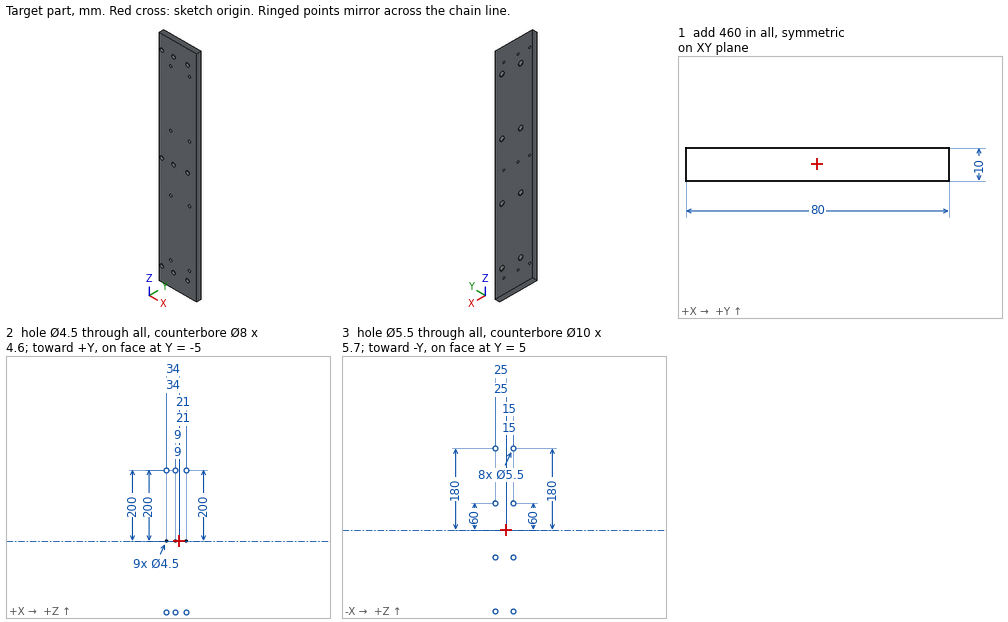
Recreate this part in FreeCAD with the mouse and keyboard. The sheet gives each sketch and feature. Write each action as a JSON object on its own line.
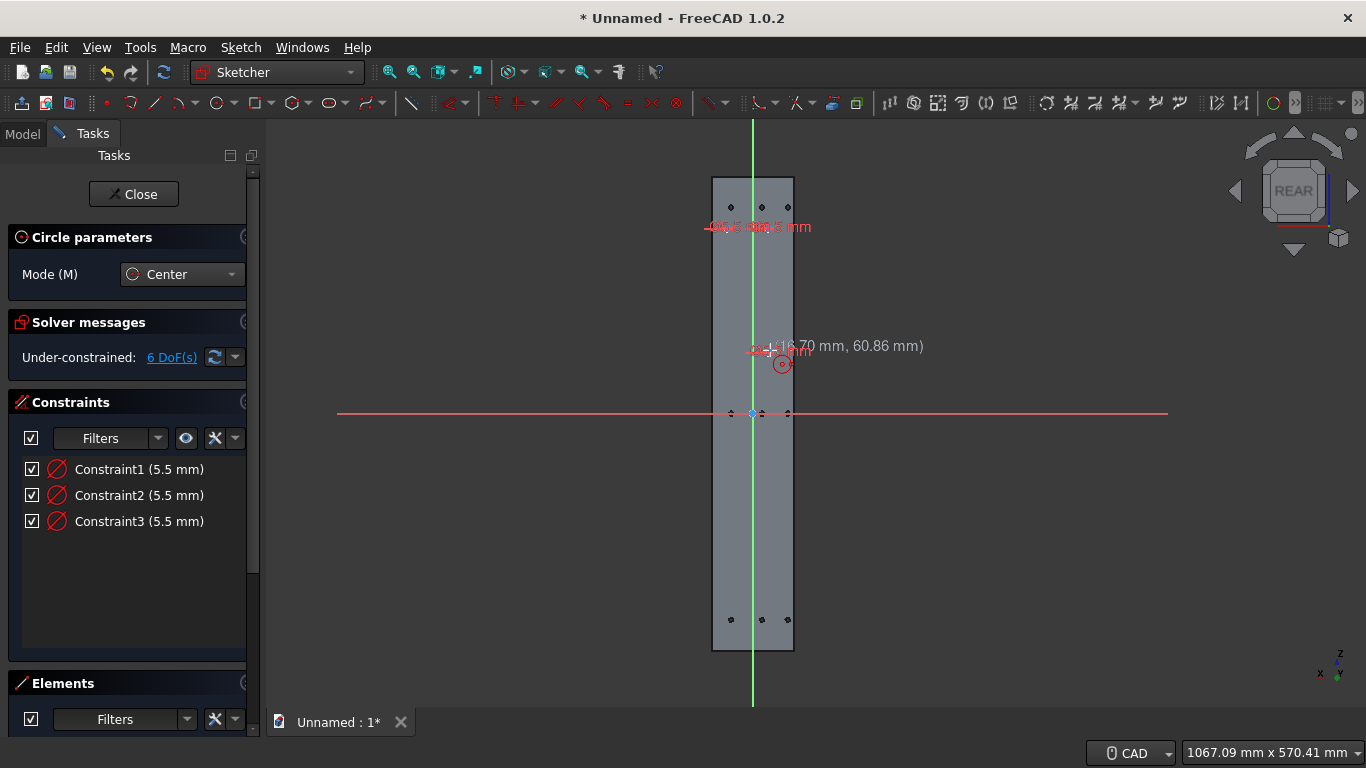
{"action": "scroll", "coordinate": [727, 352], "scroll_direction": "up", "scroll_amount": 11}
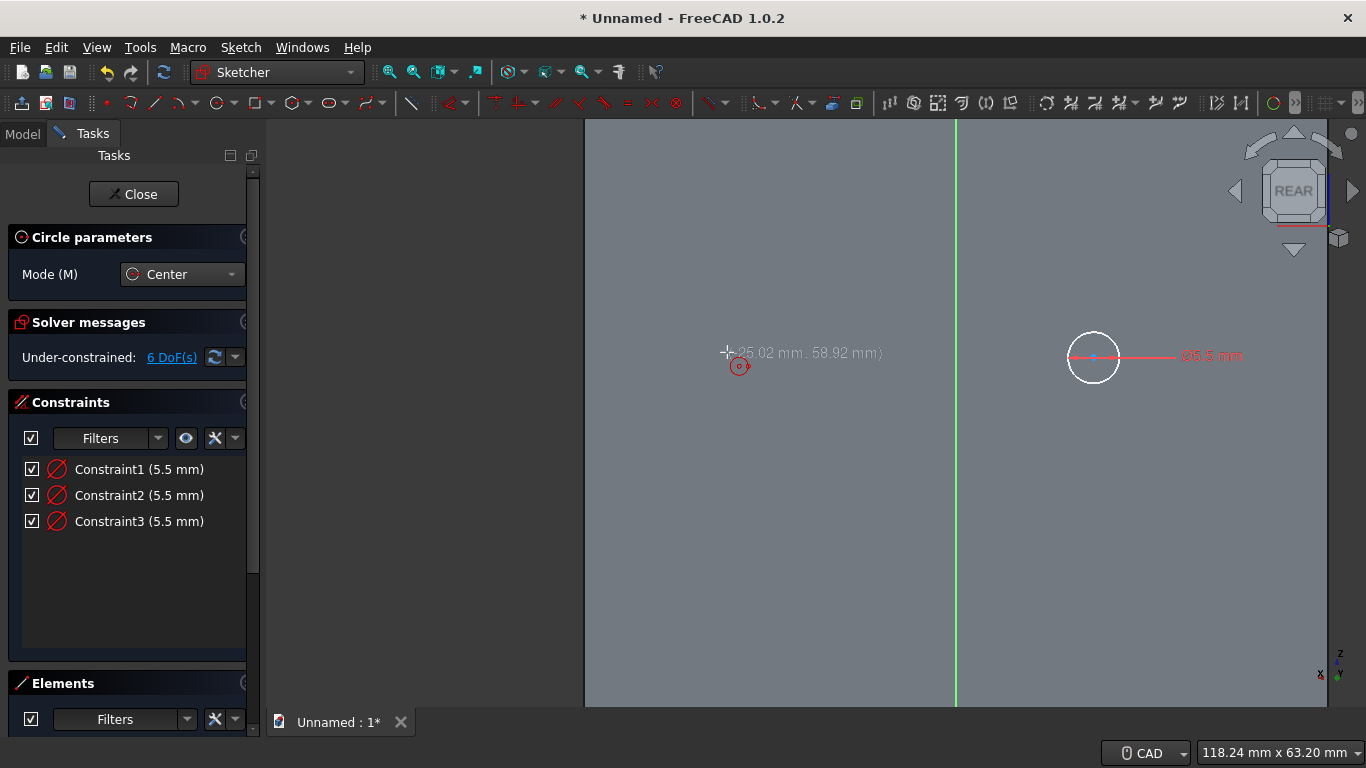
{"action": "scroll", "coordinate": [727, 352], "scroll_direction": "down", "scroll_amount": 11}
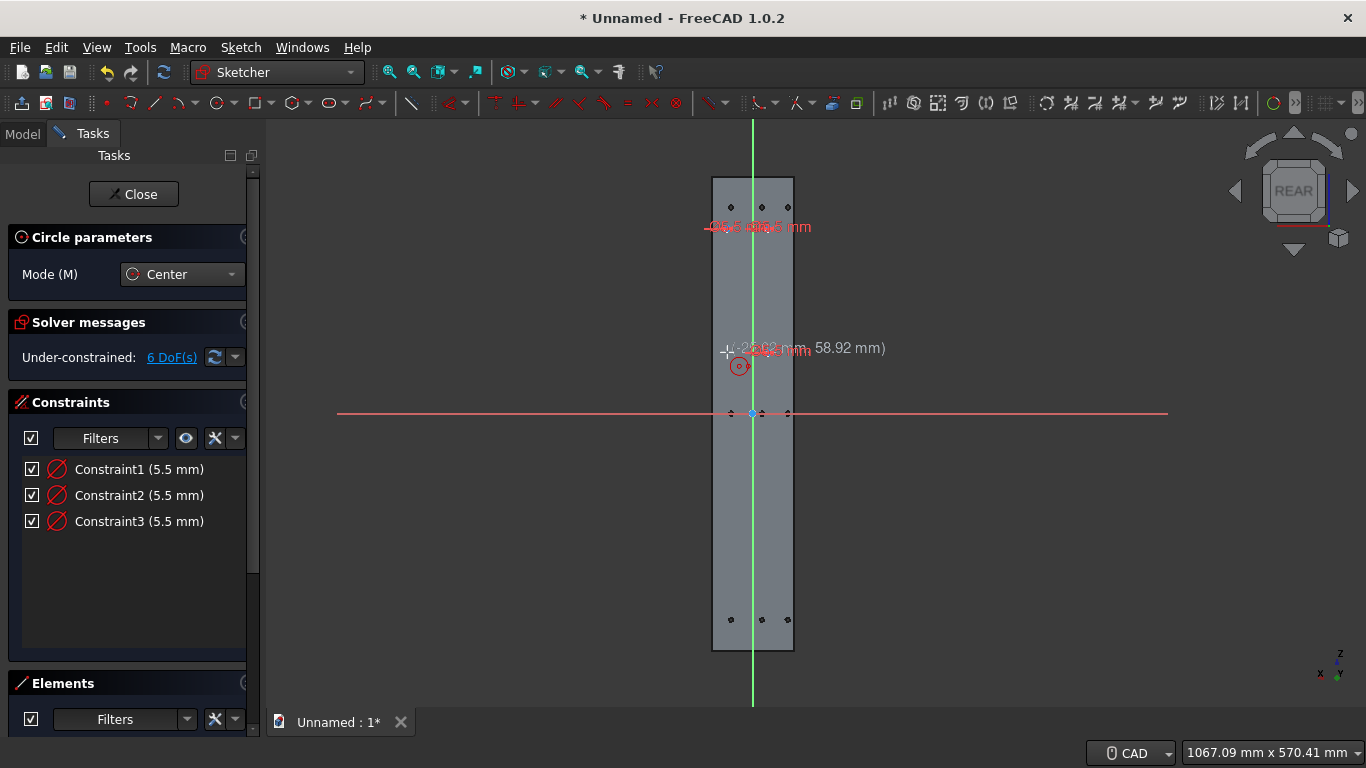
{"action": "left_click", "coordinate": [727, 352]}
{"action": "mouse_move", "coordinate": [729, 350]}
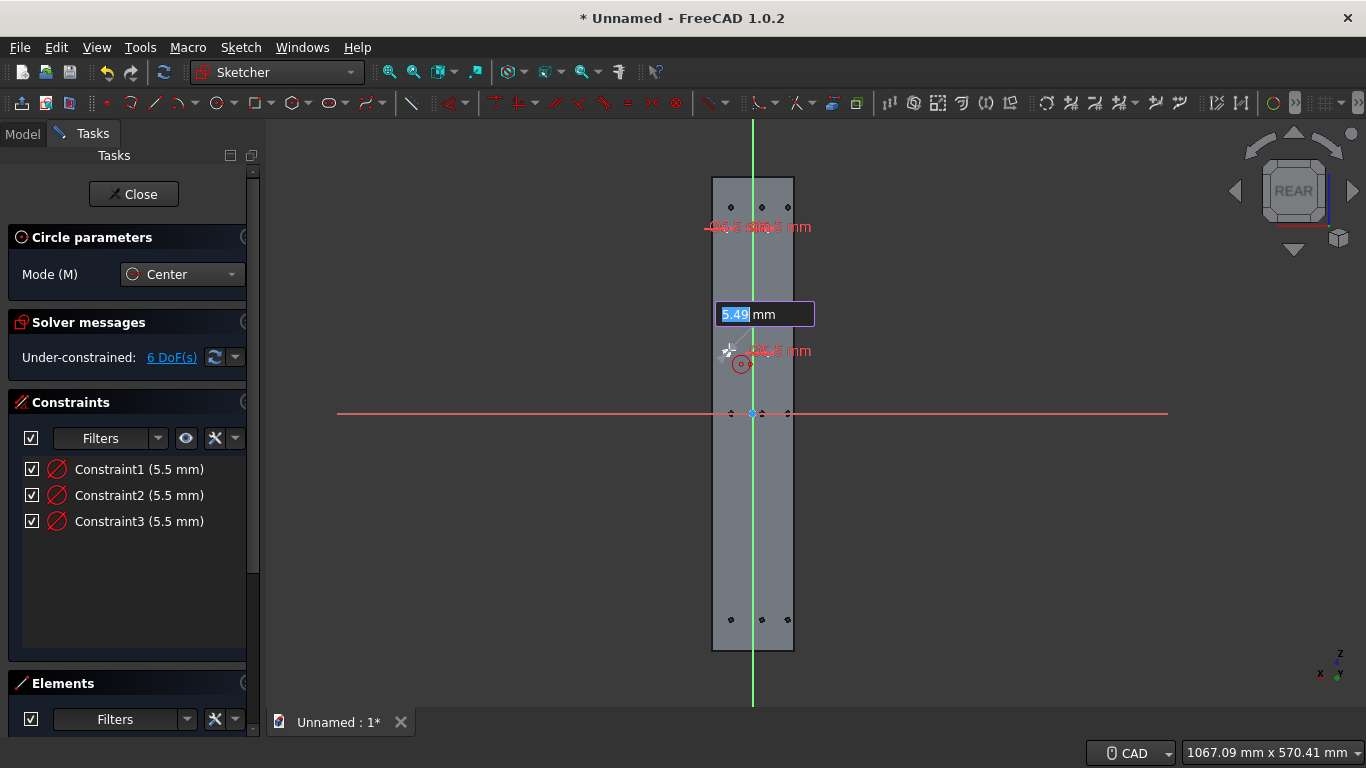
{"action": "type", "text": "5.5"}
{"action": "key", "text": "Return"}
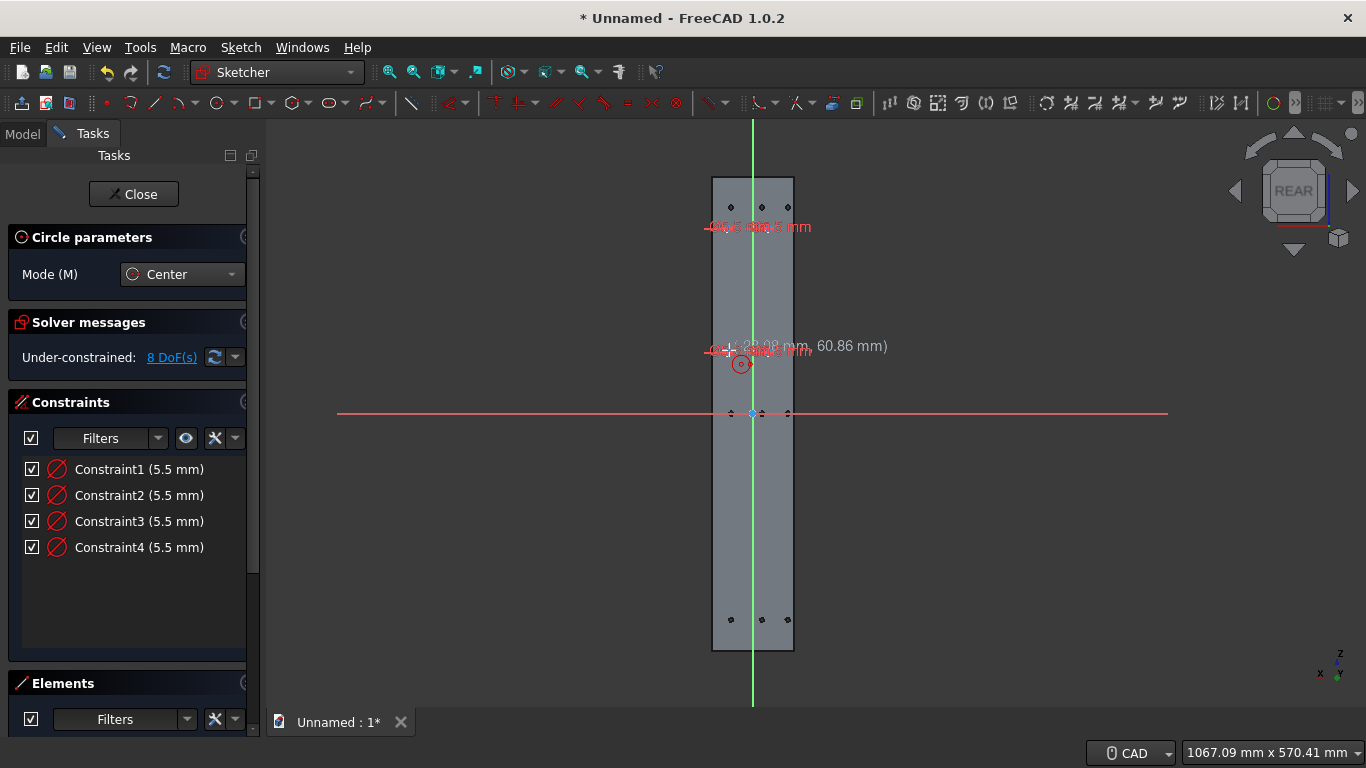
{"action": "scroll", "coordinate": [727, 476], "scroll_direction": "up", "scroll_amount": 11}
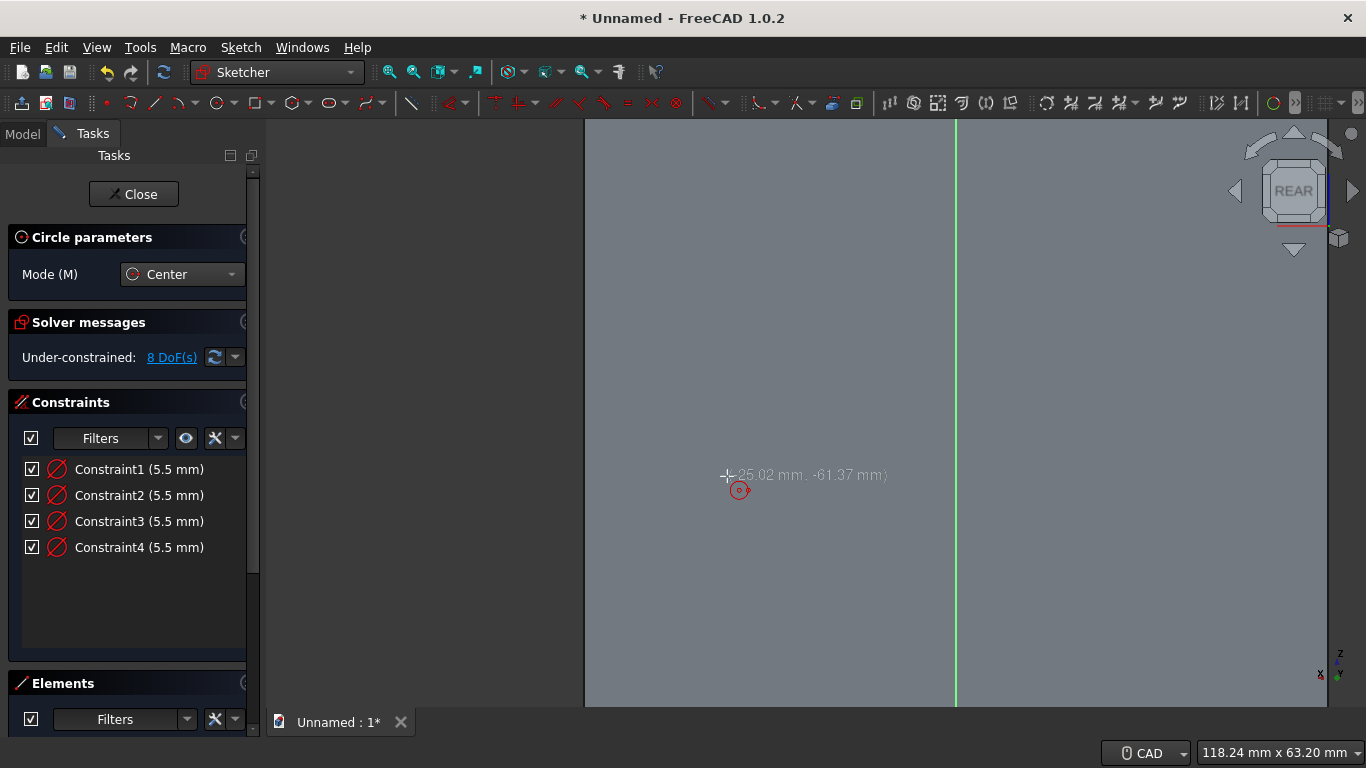
{"action": "scroll", "coordinate": [727, 476], "scroll_direction": "down", "scroll_amount": 11}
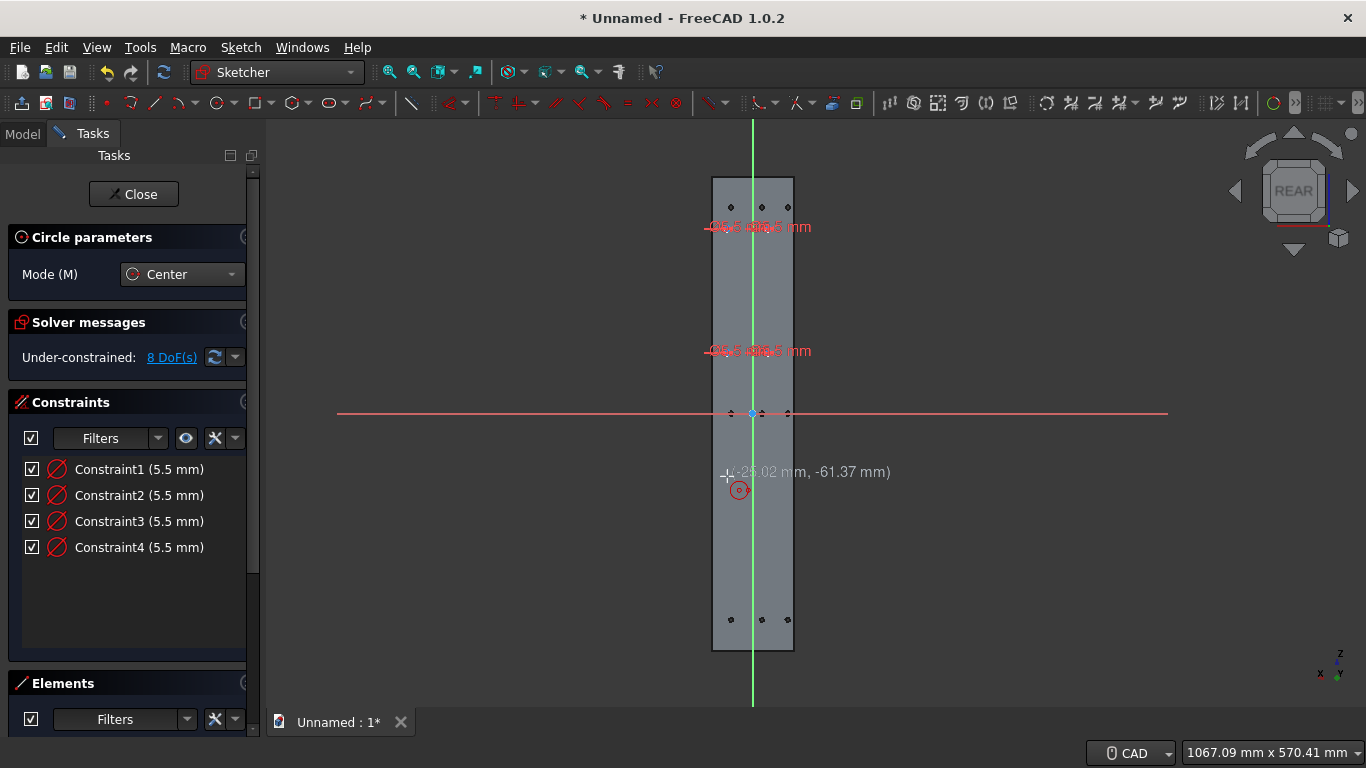
{"action": "left_click", "coordinate": [727, 476]}
{"action": "mouse_move", "coordinate": [729, 474]}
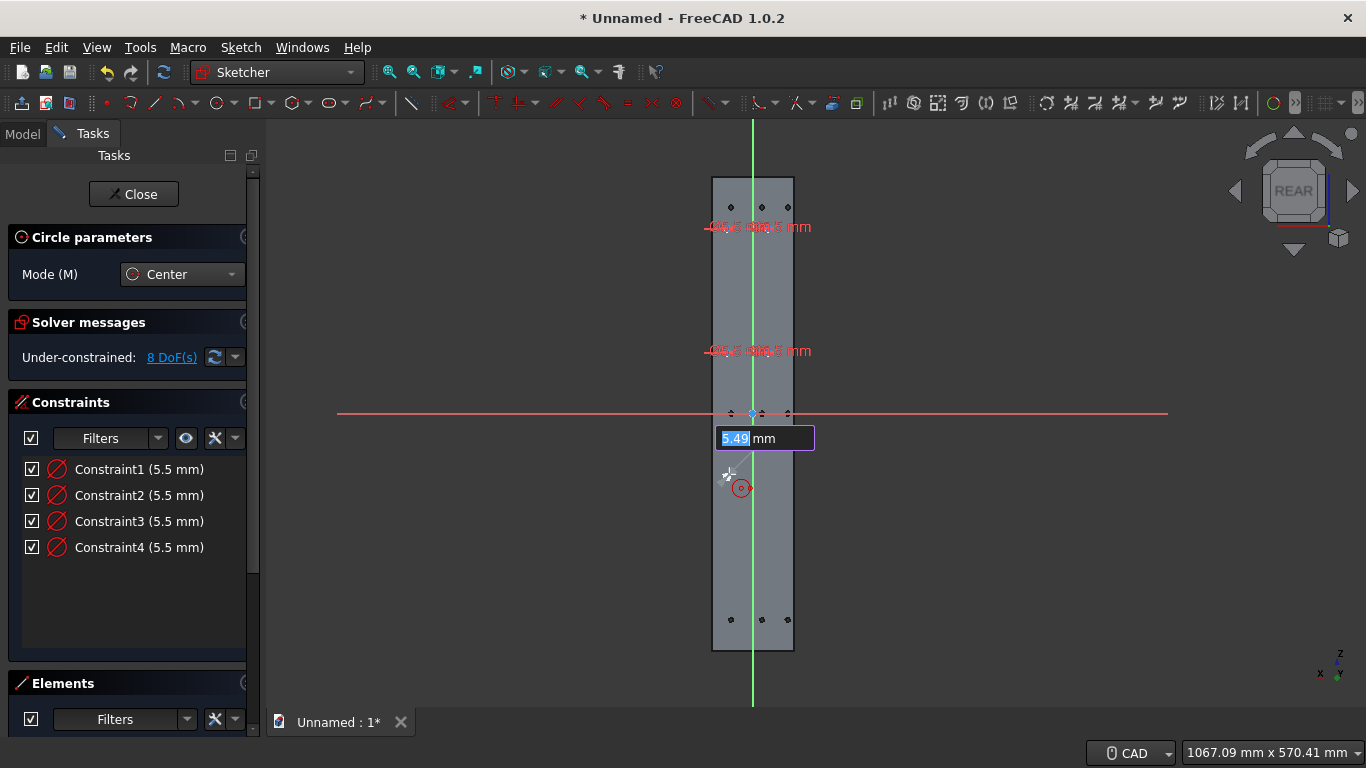
{"action": "type", "text": "5.5"}
{"action": "key", "text": "Return"}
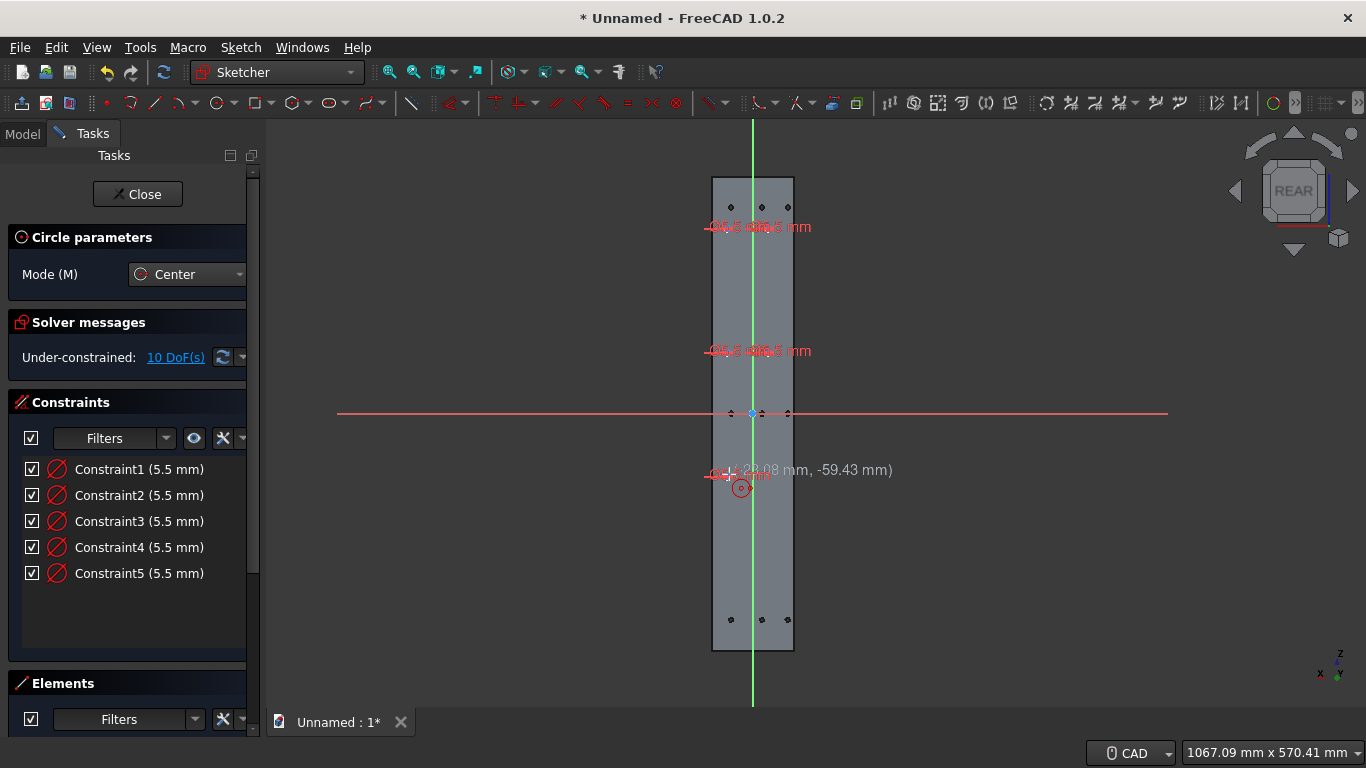
{"action": "scroll", "coordinate": [727, 599], "scroll_direction": "up", "scroll_amount": 11}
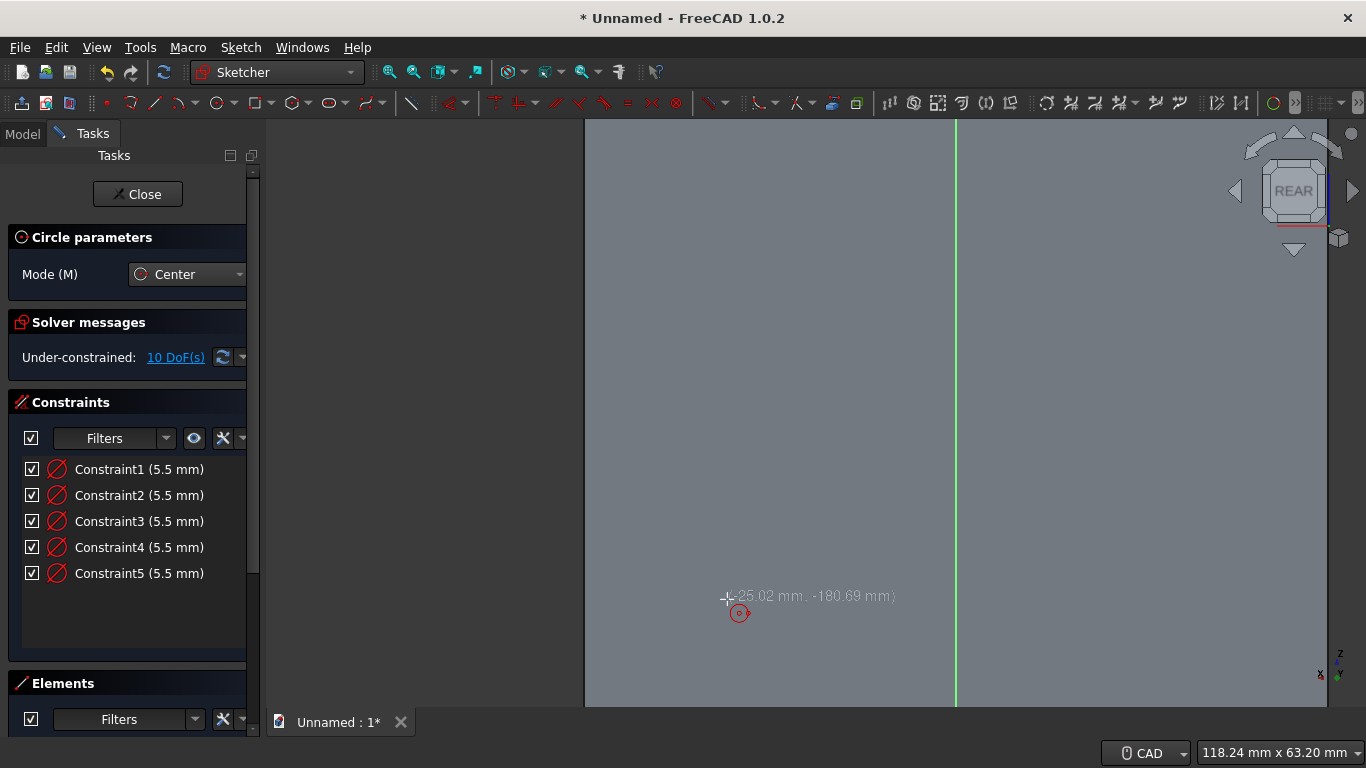
{"action": "scroll", "coordinate": [727, 599], "scroll_direction": "down", "scroll_amount": 11}